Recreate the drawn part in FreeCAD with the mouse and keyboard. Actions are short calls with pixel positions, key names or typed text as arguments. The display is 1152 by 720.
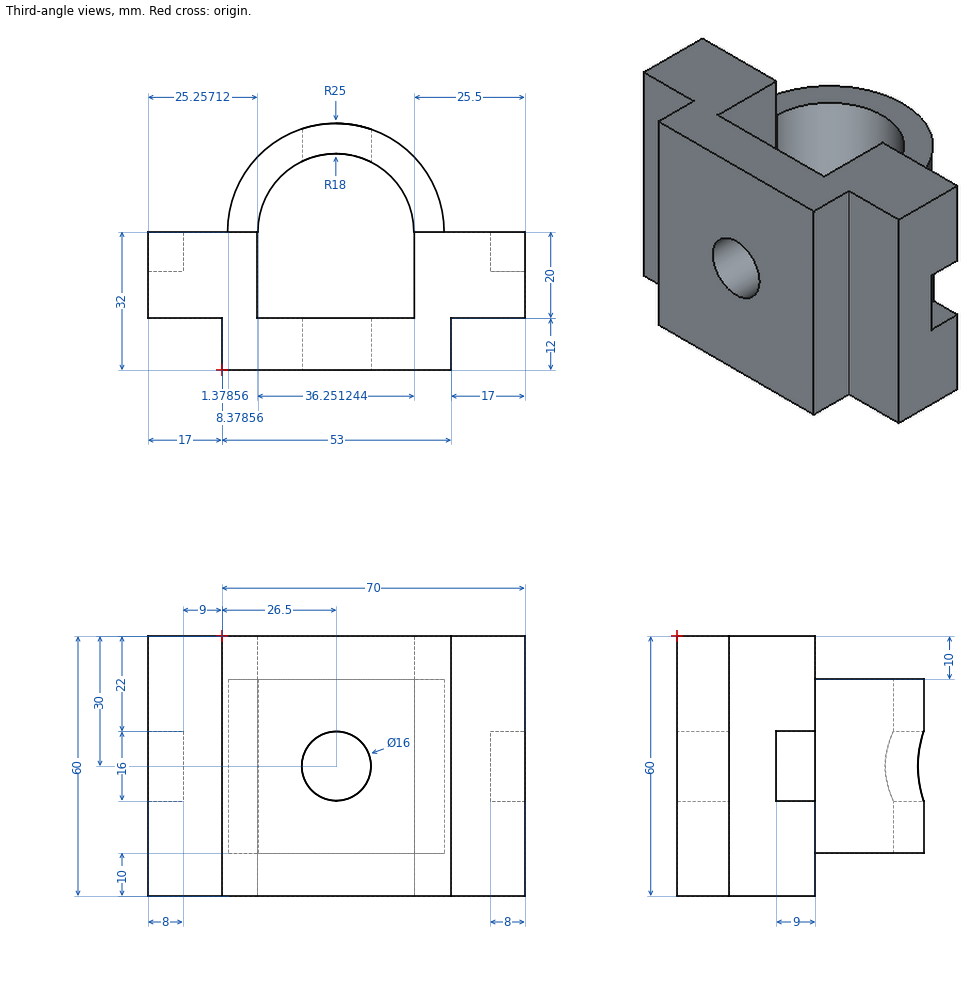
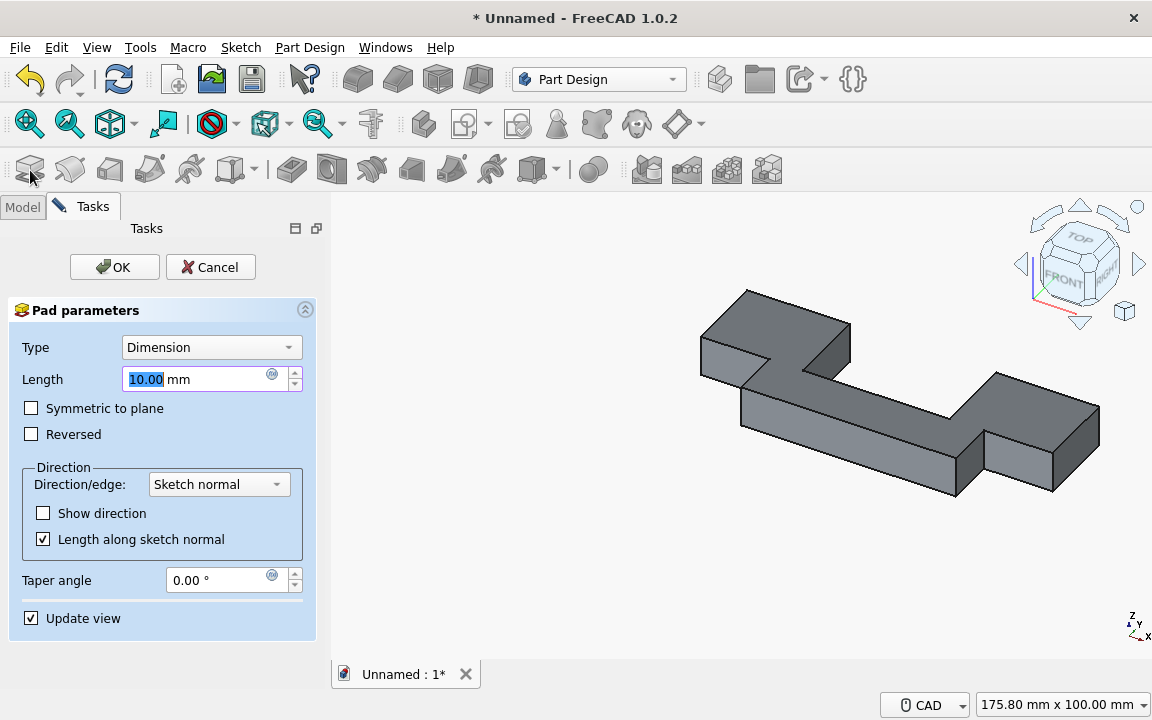
text(60)
key(Tab)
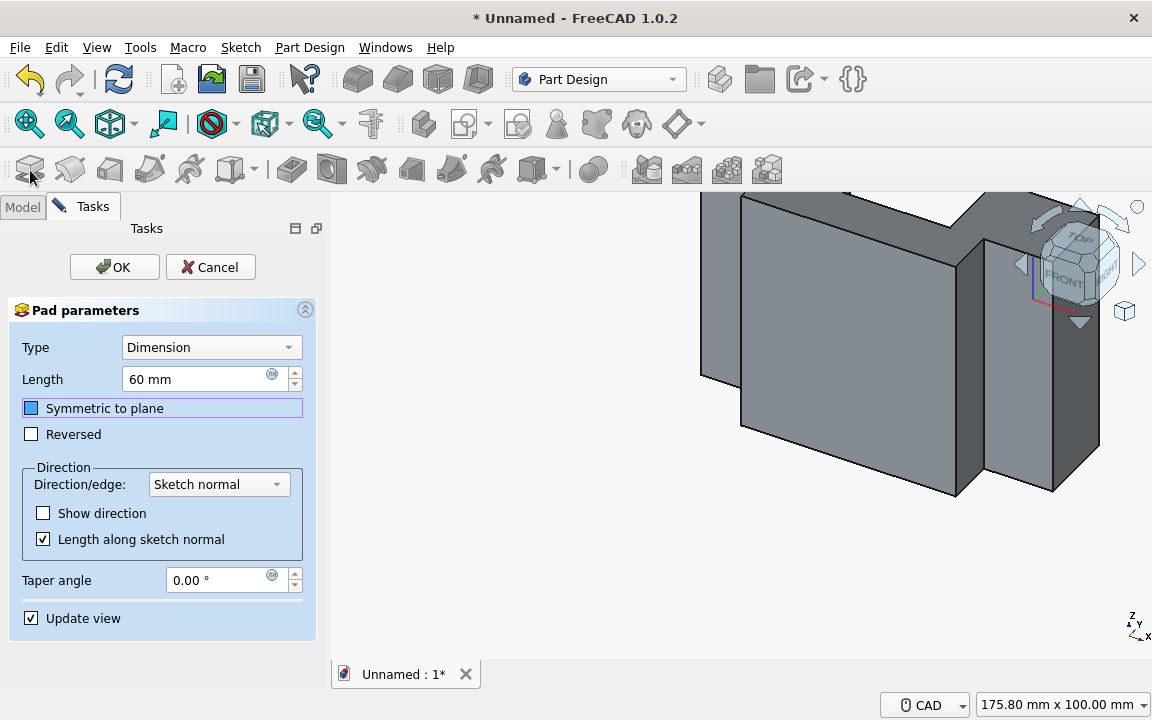
click(30, 434)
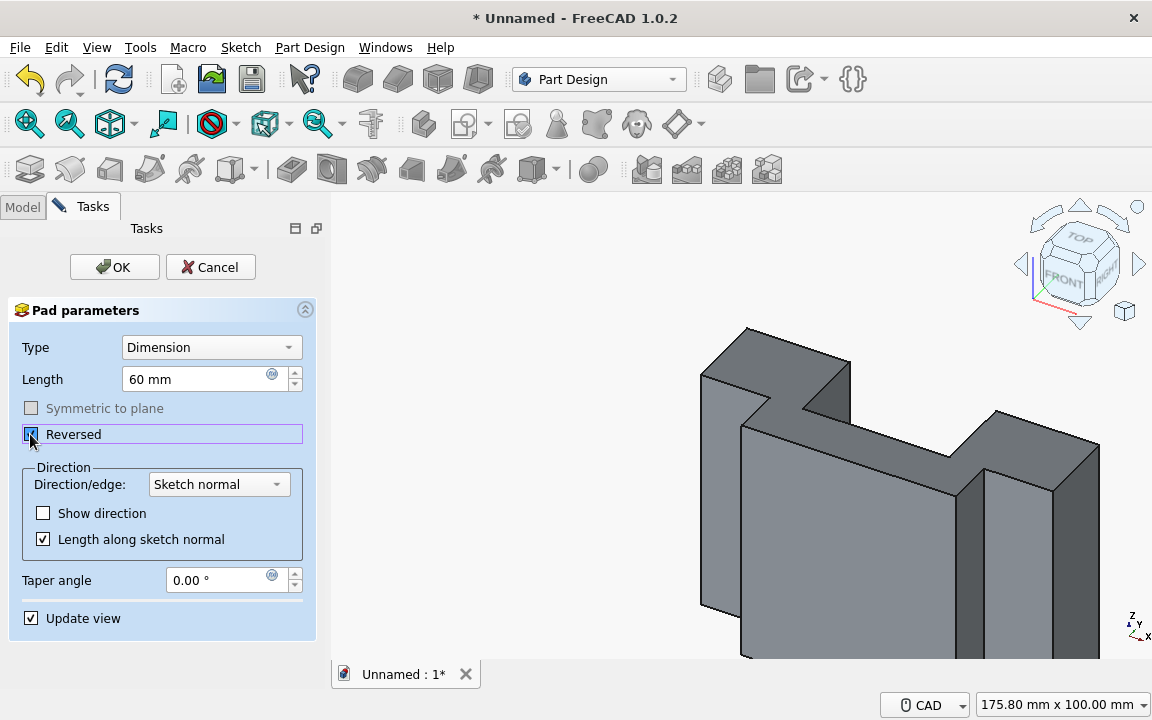
click(115, 267)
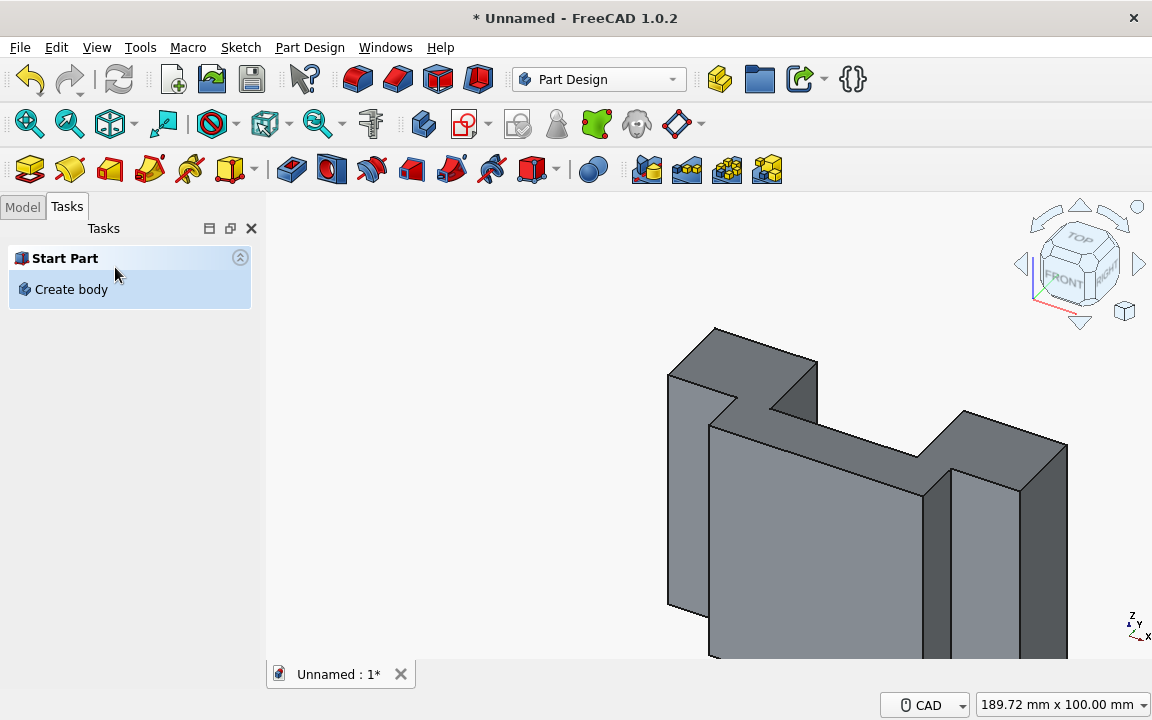
key(v)
key(f)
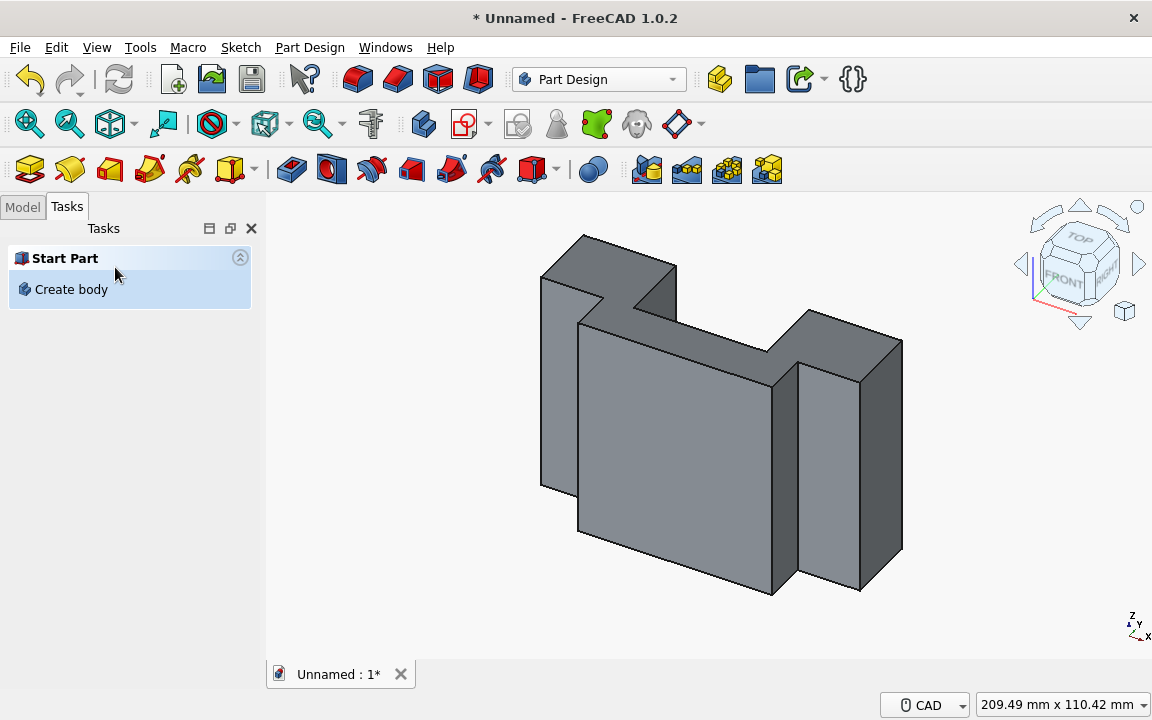
click(819, 332)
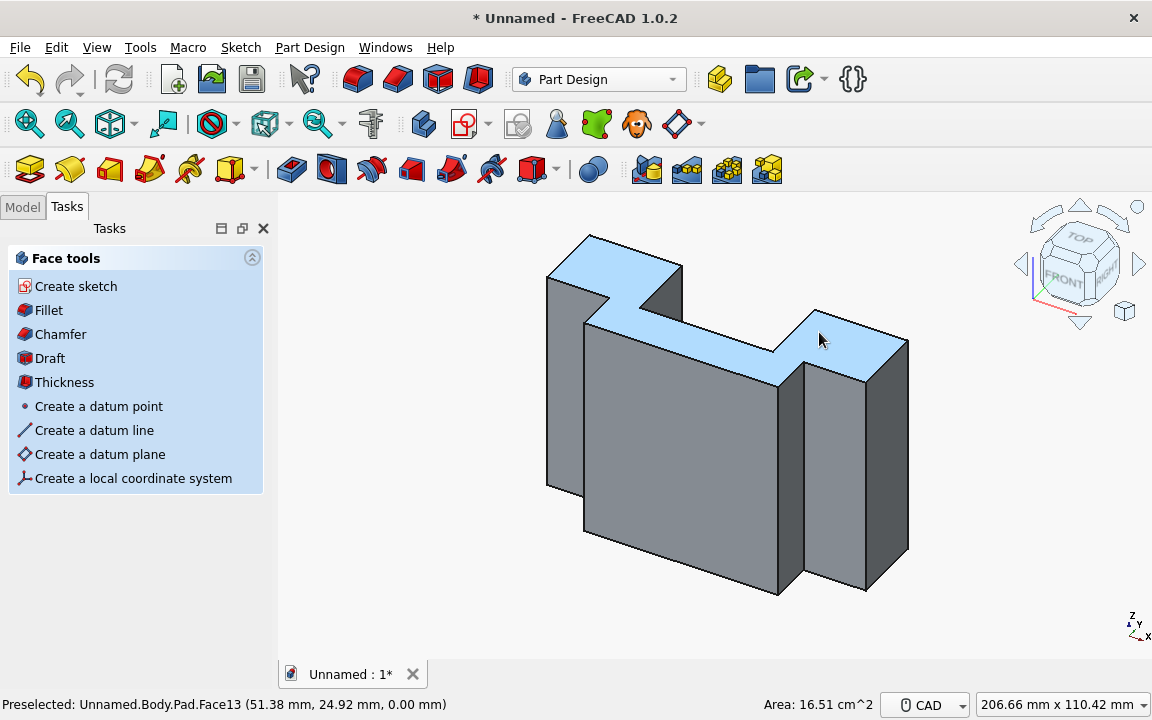
click(464, 124)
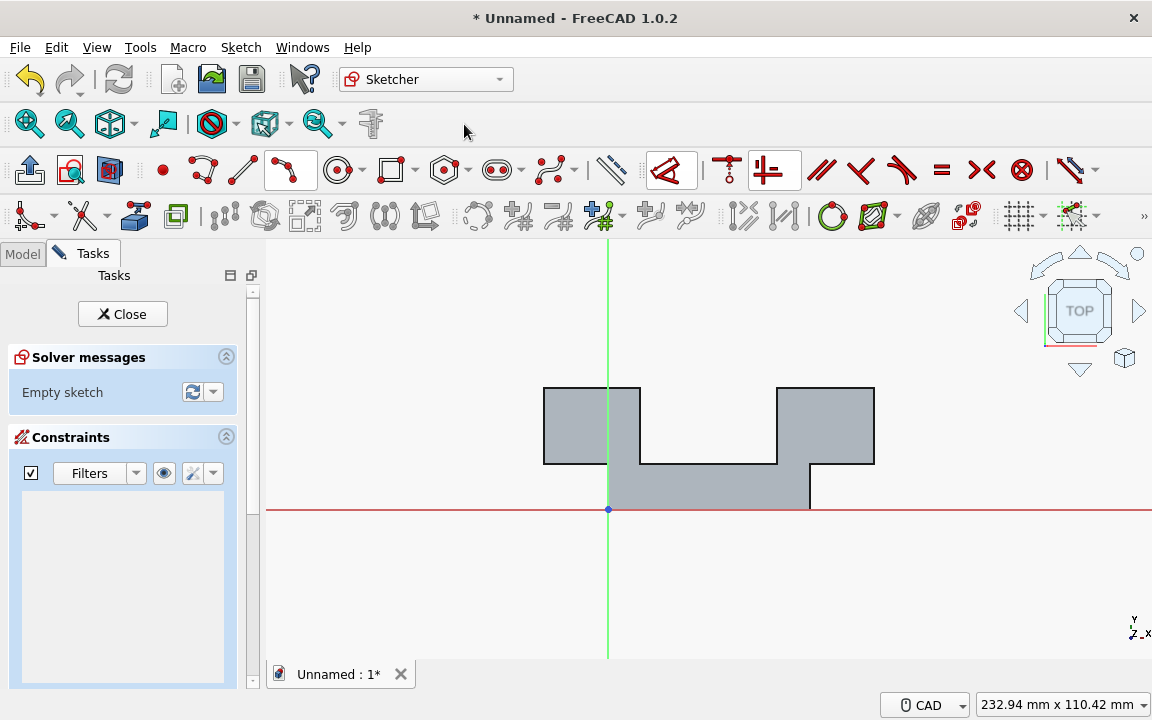
key(g)
key(l)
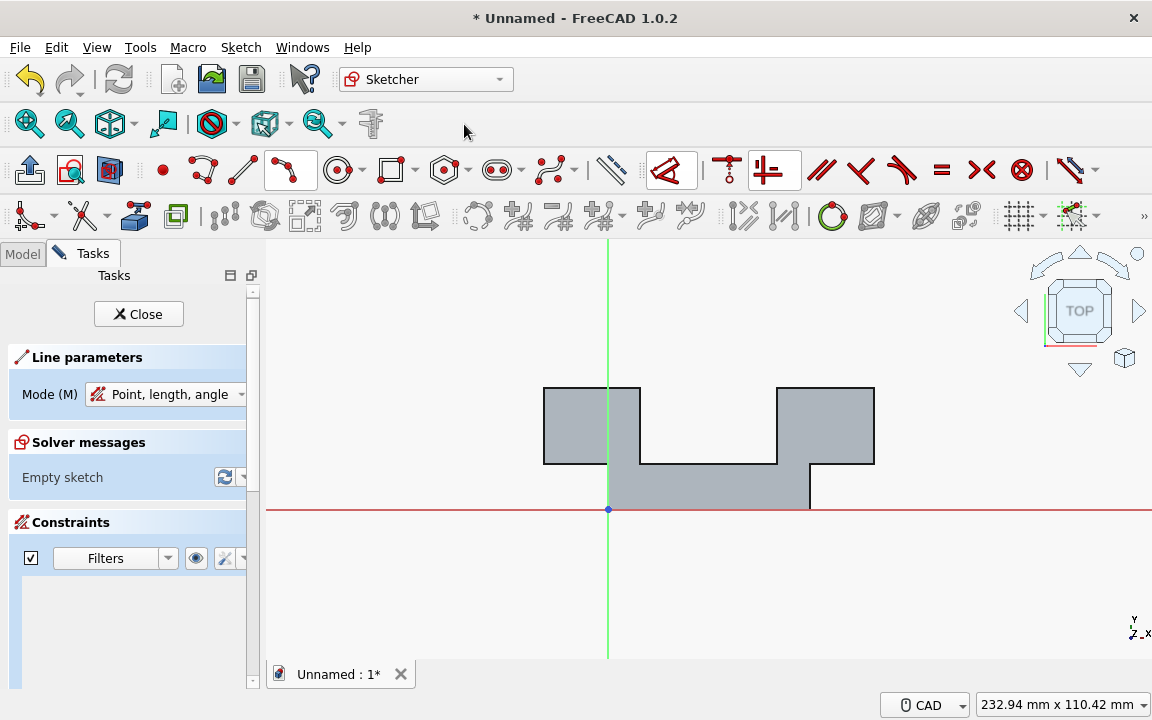
scroll(613, 388, up, 6)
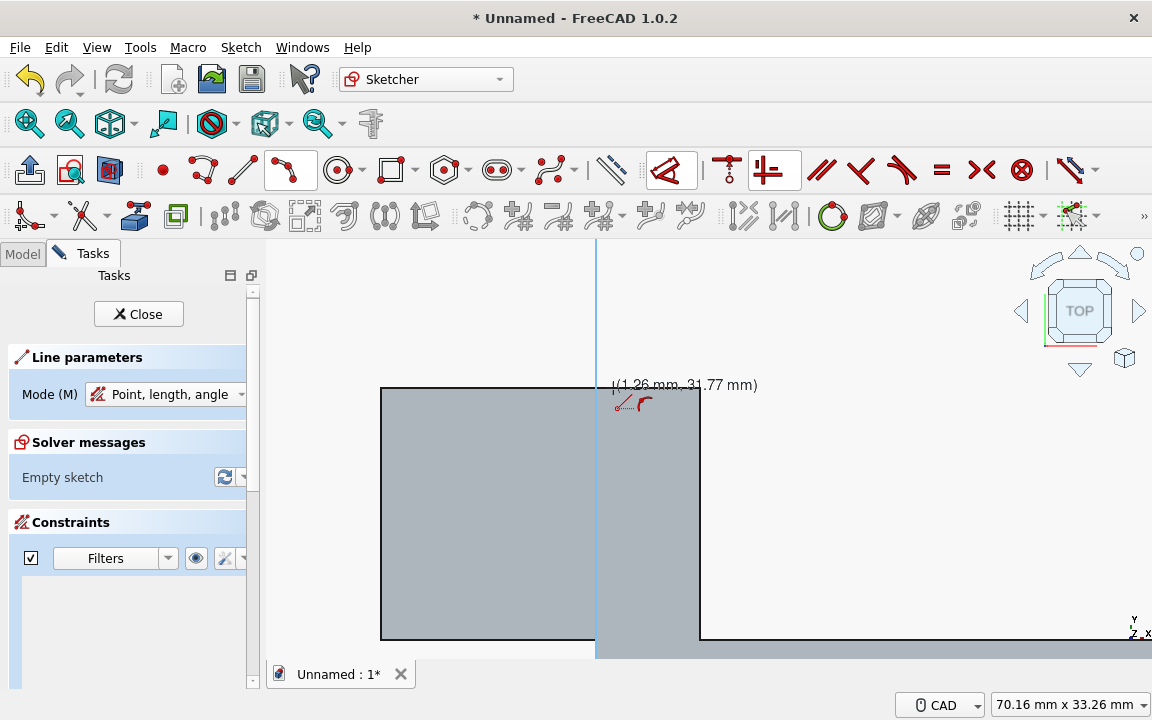
click(614, 388)
click(702, 388)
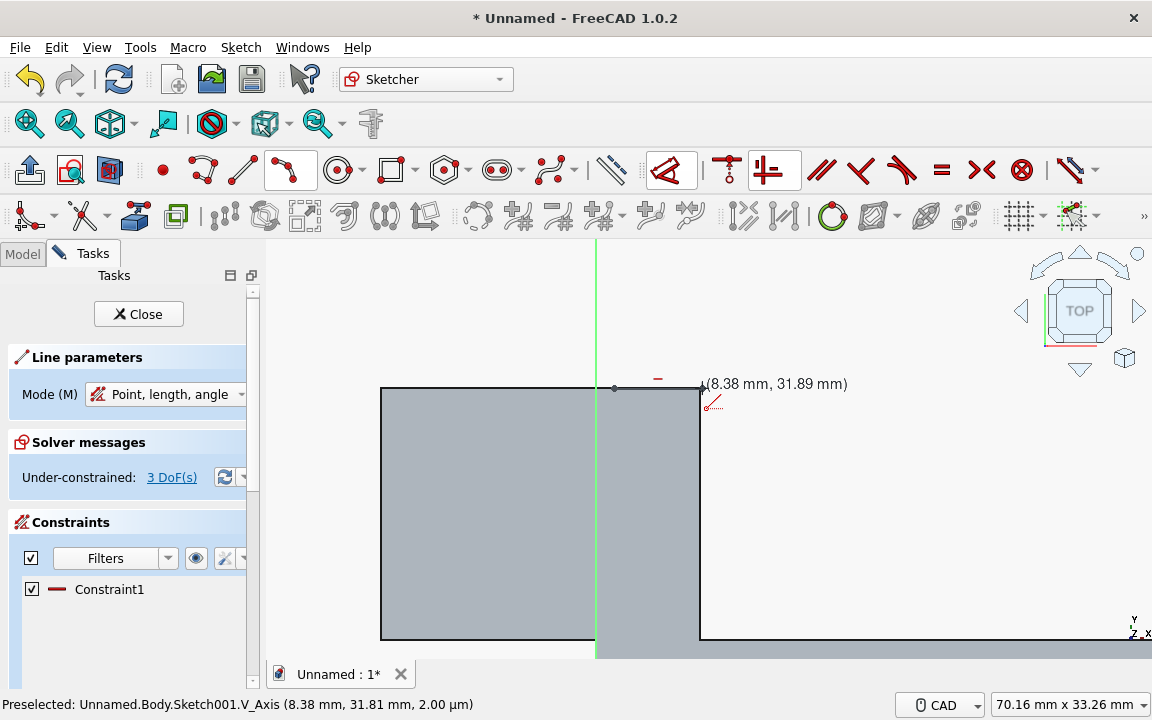
scroll(477, 459, down, 5)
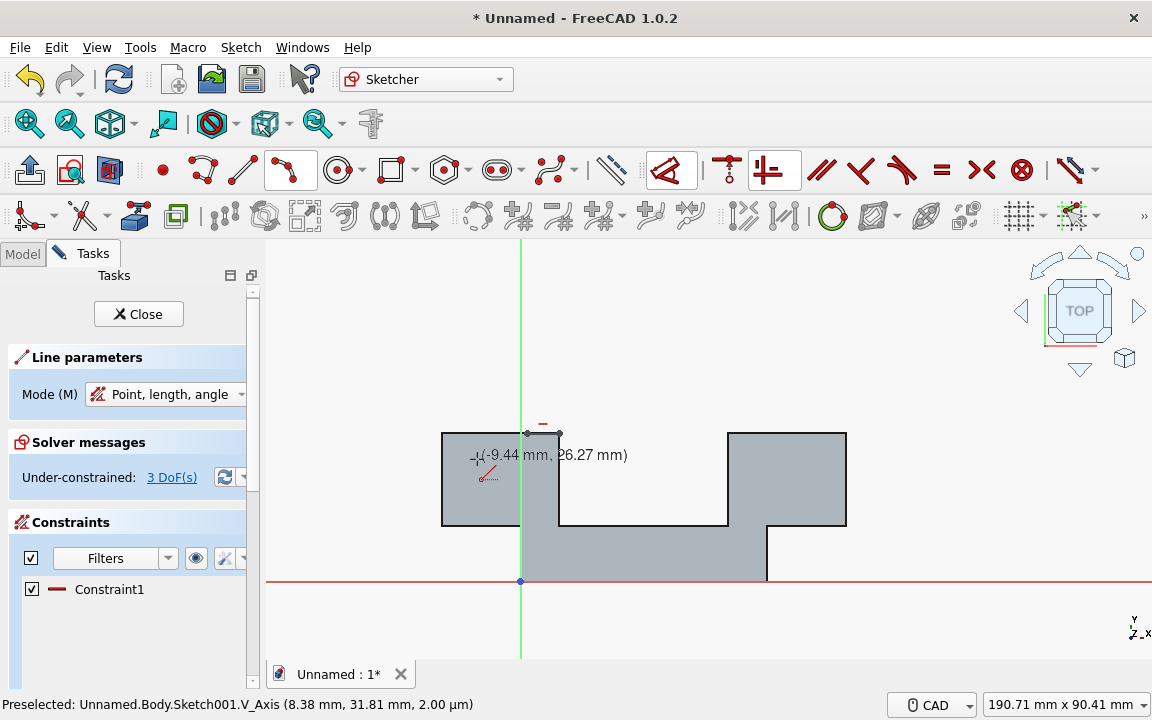
click(727, 433)
click(760, 433)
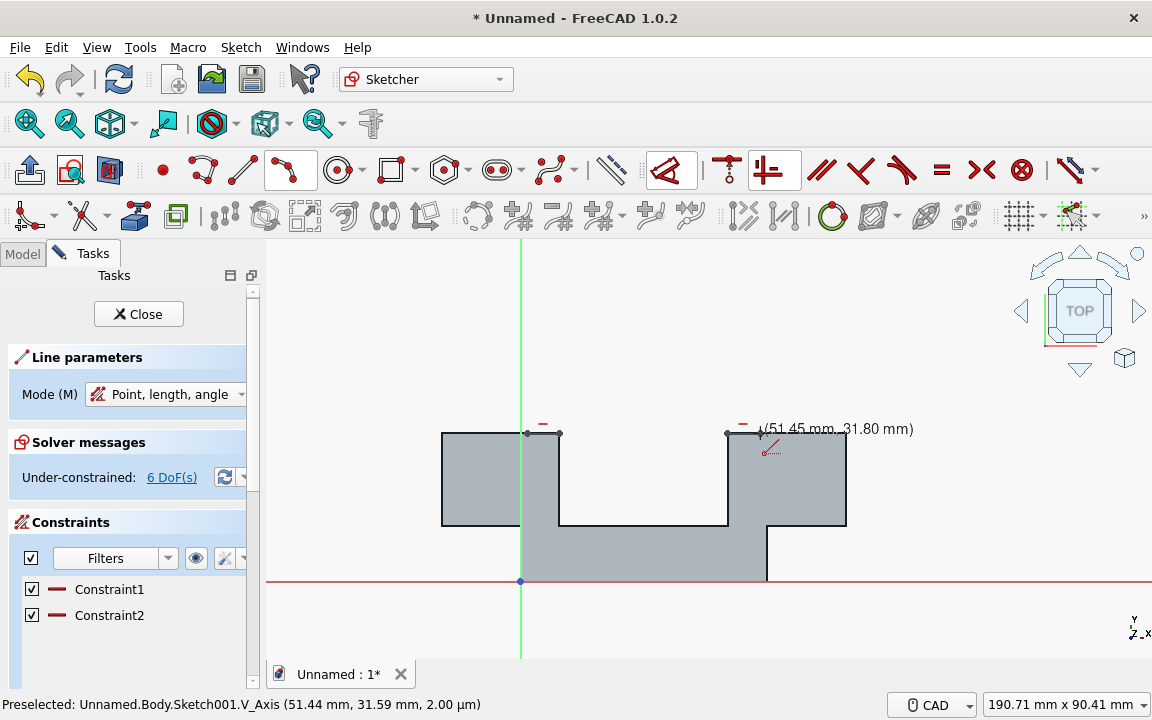
key(g)
key(3)
key(a)